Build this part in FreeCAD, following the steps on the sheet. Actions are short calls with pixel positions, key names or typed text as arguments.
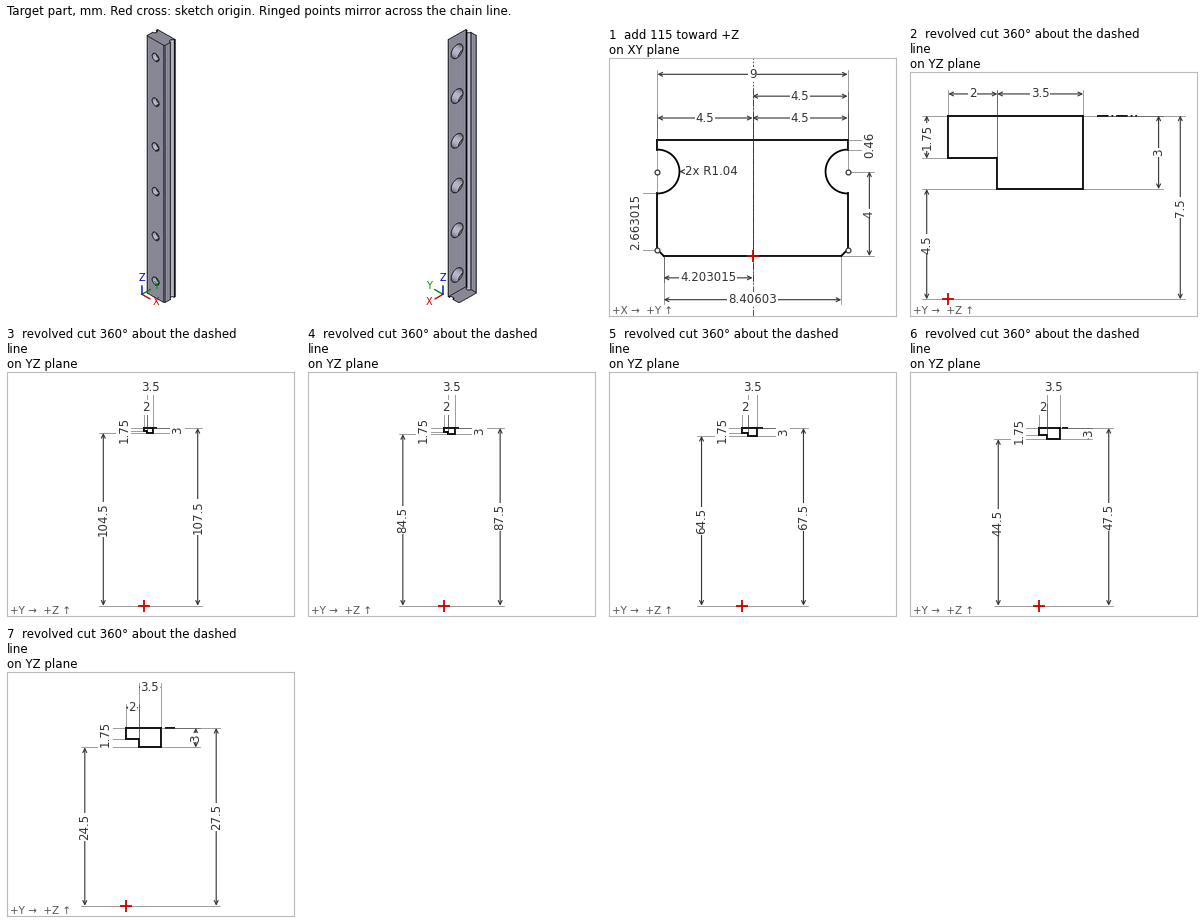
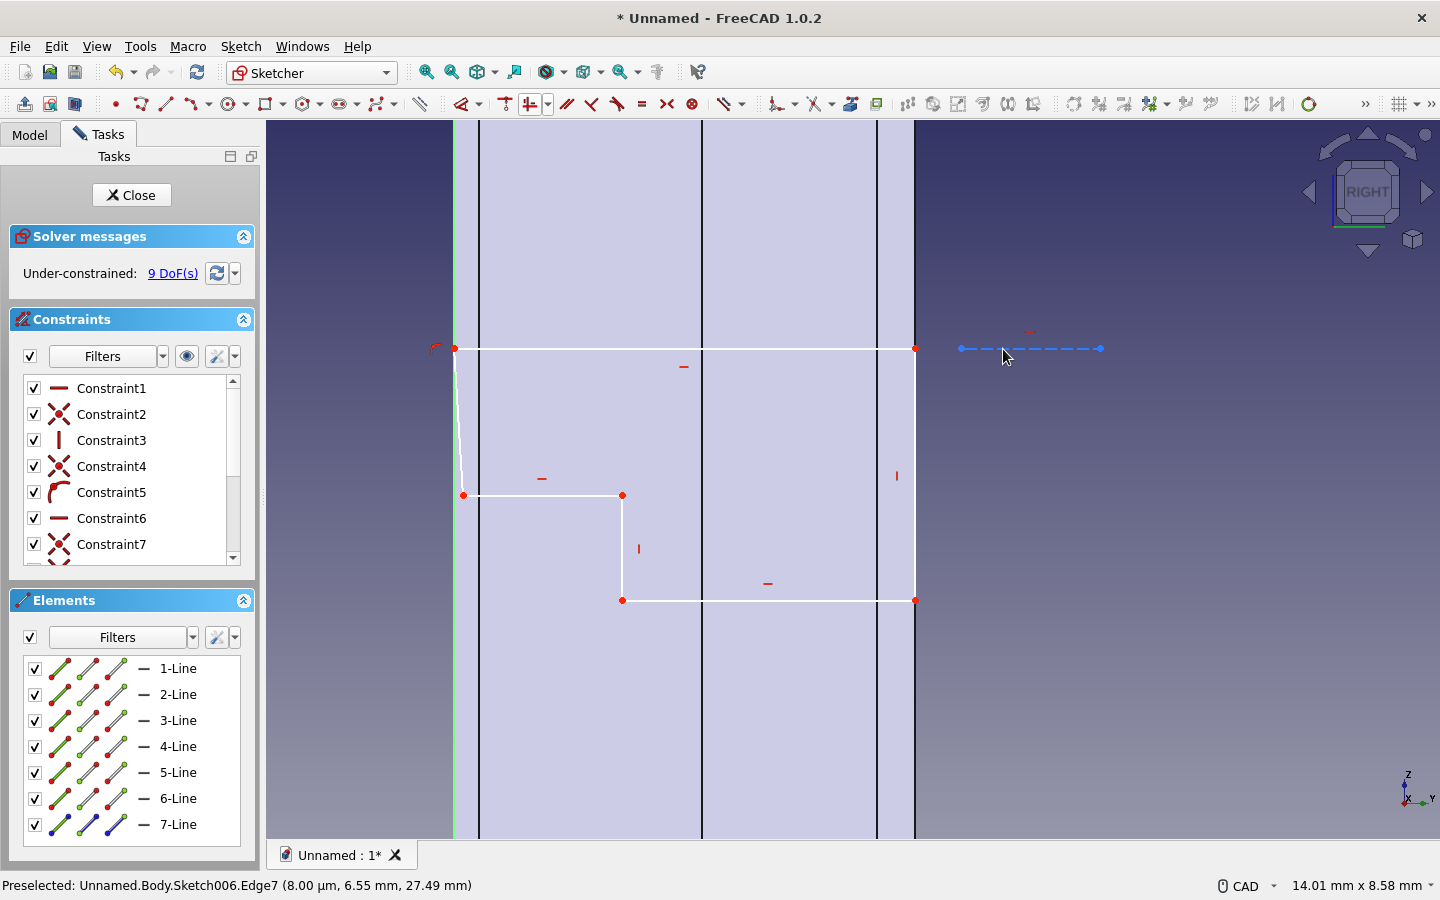
click(457, 393)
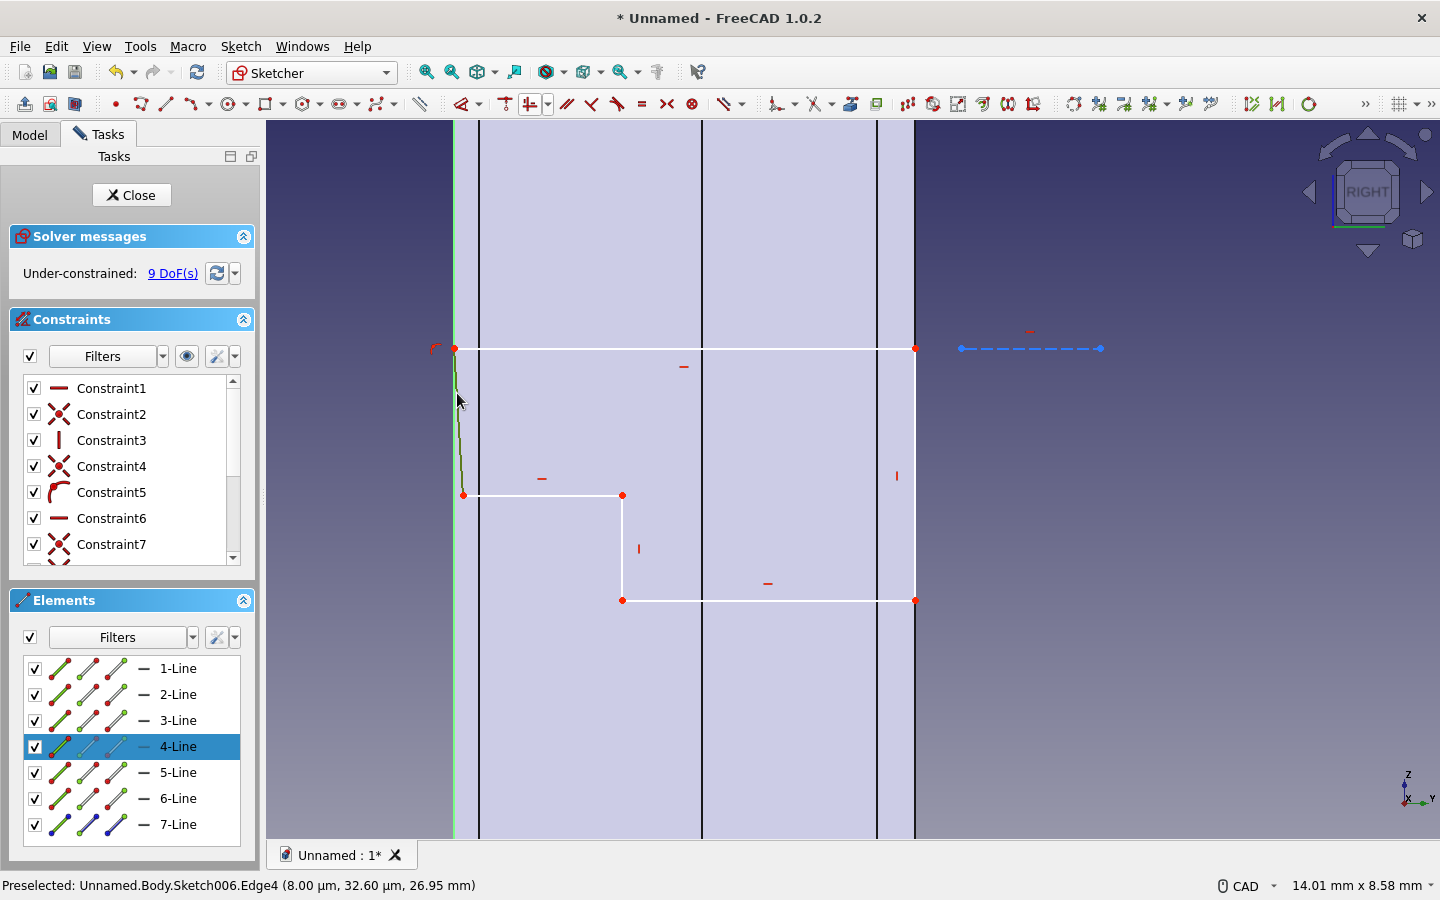
key(v)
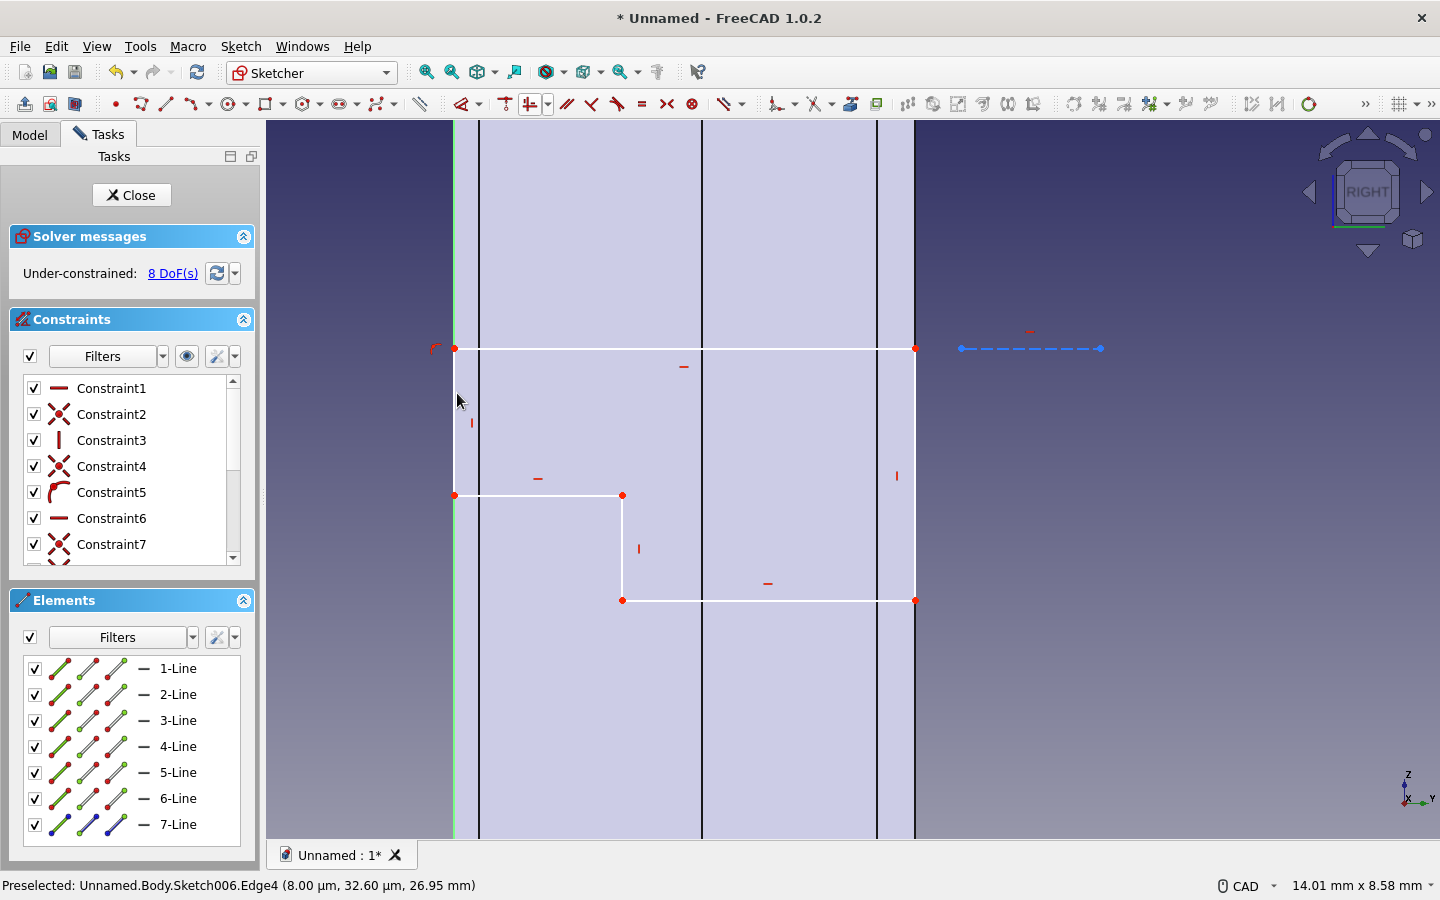
key(d)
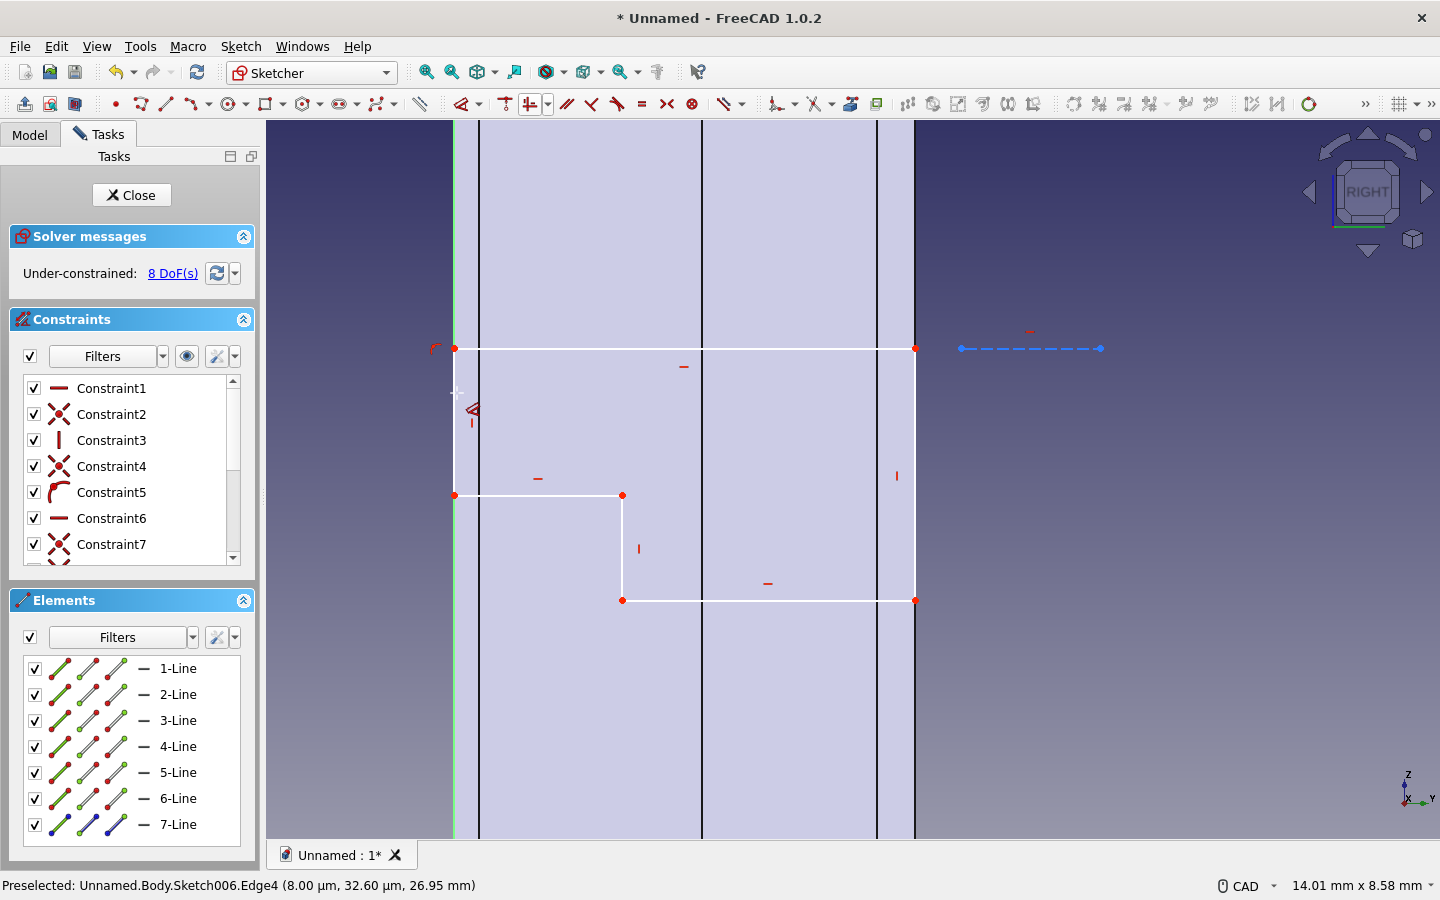
click(915, 525)
click(949, 475)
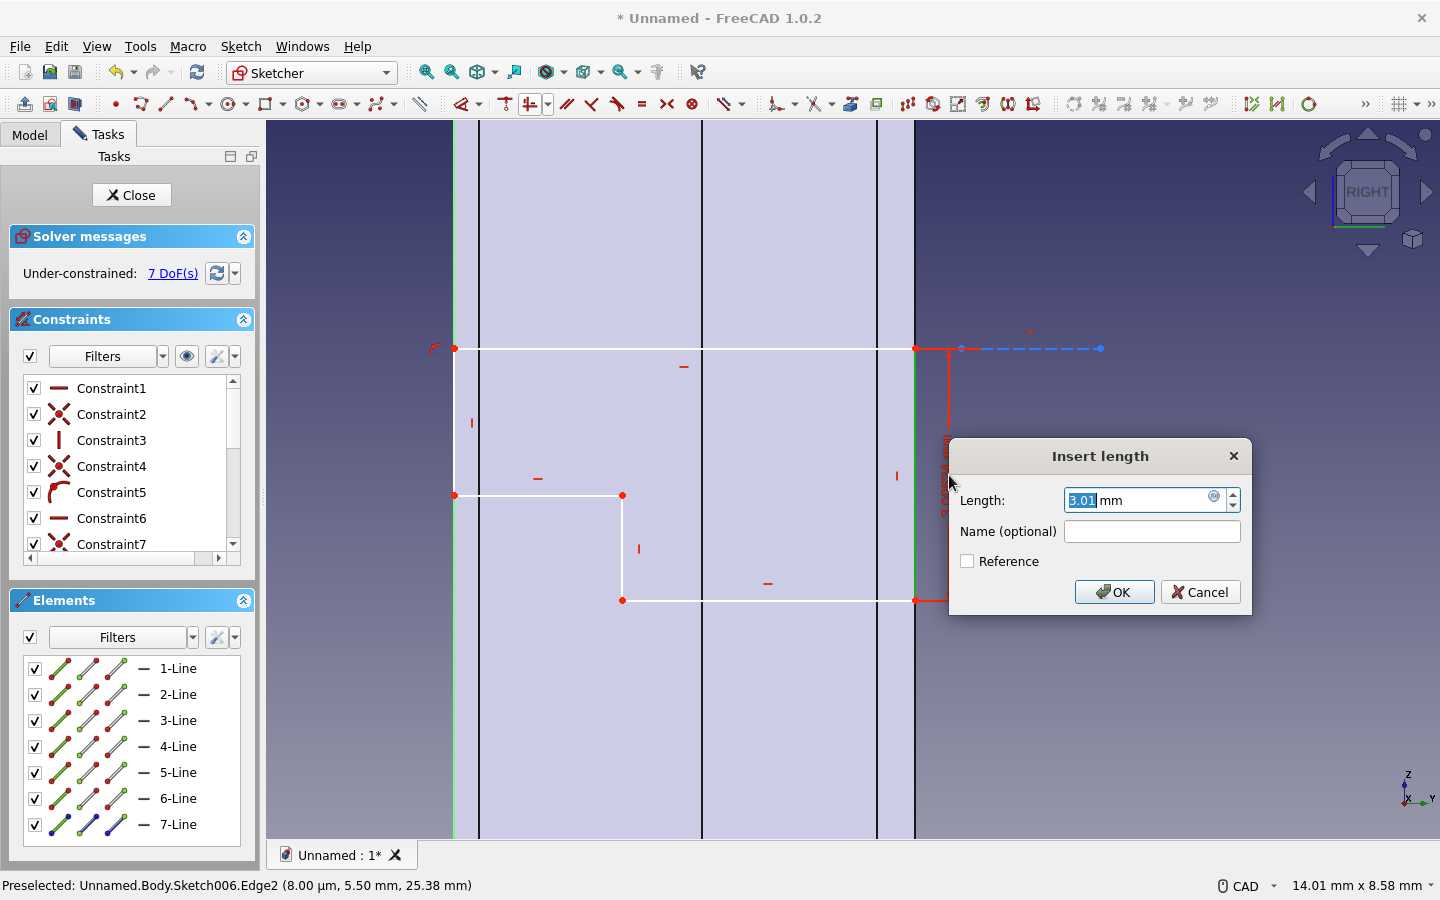
text(3)
key(Return)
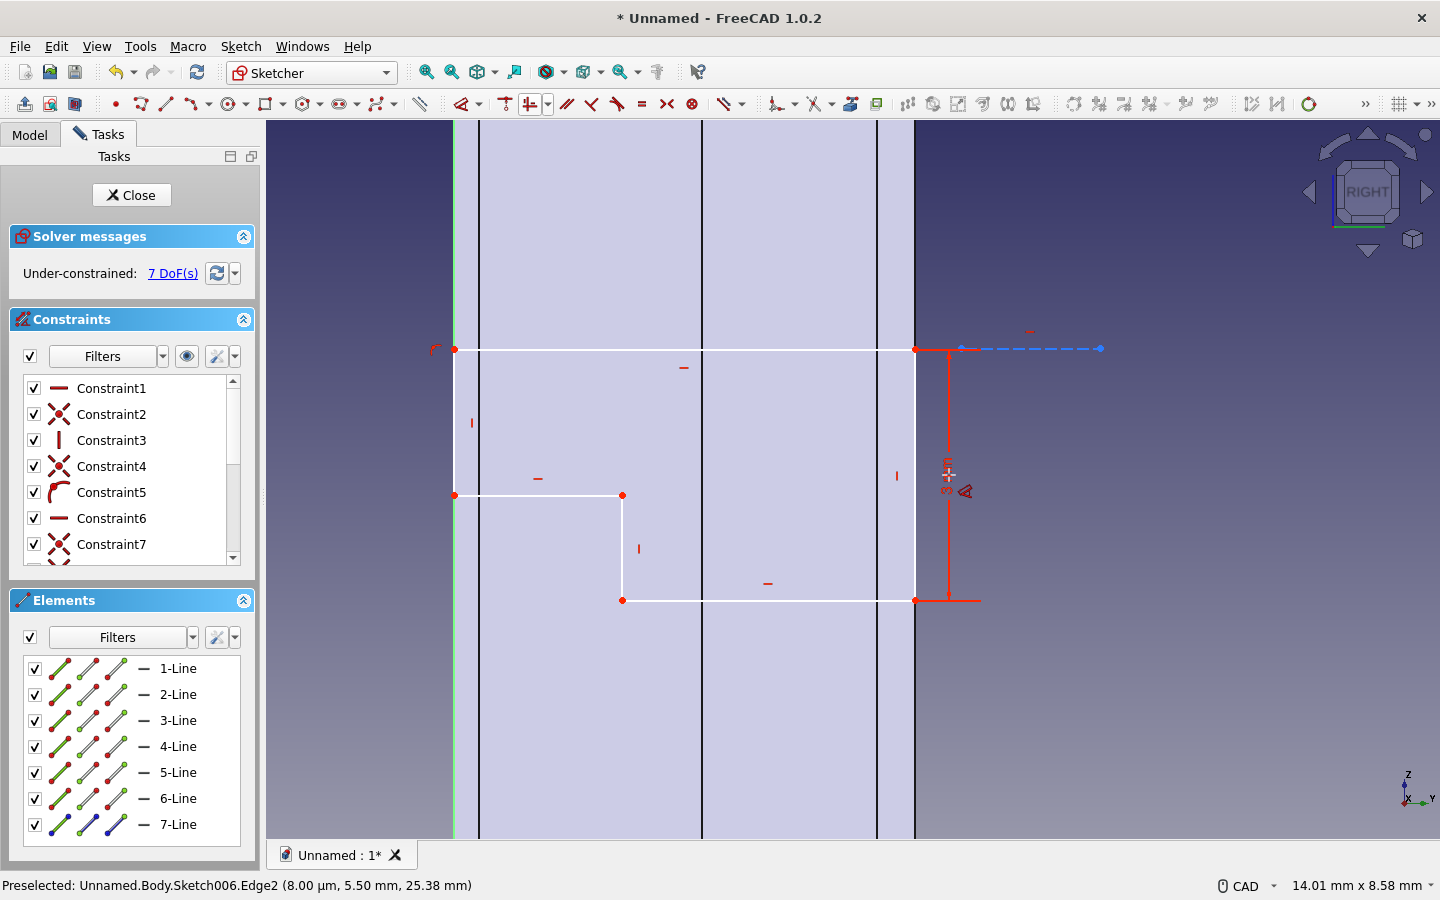
click(504, 496)
click(538, 530)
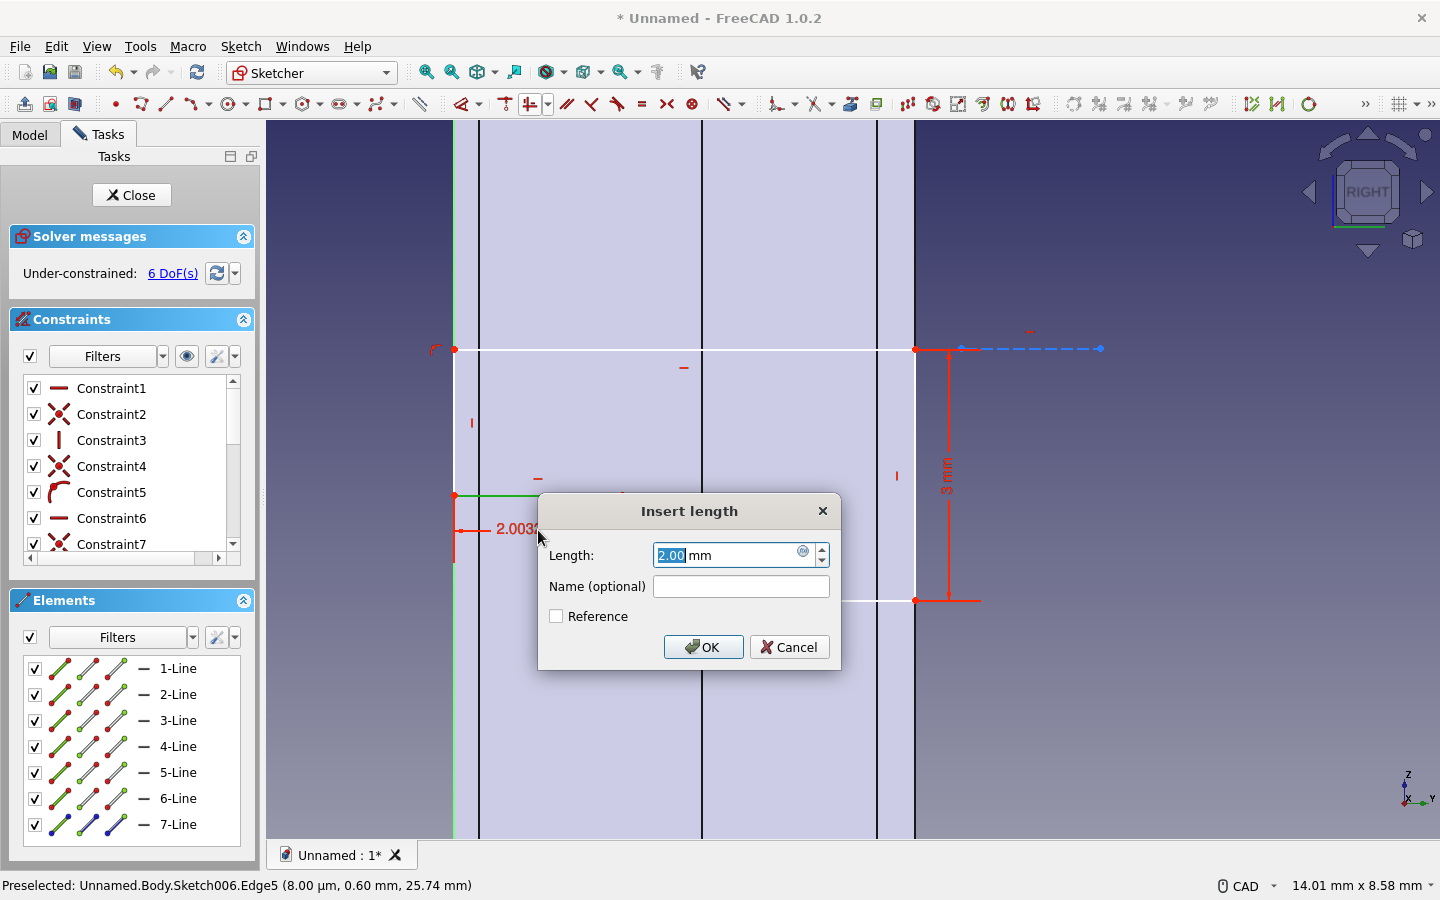
text(2)
key(Return)